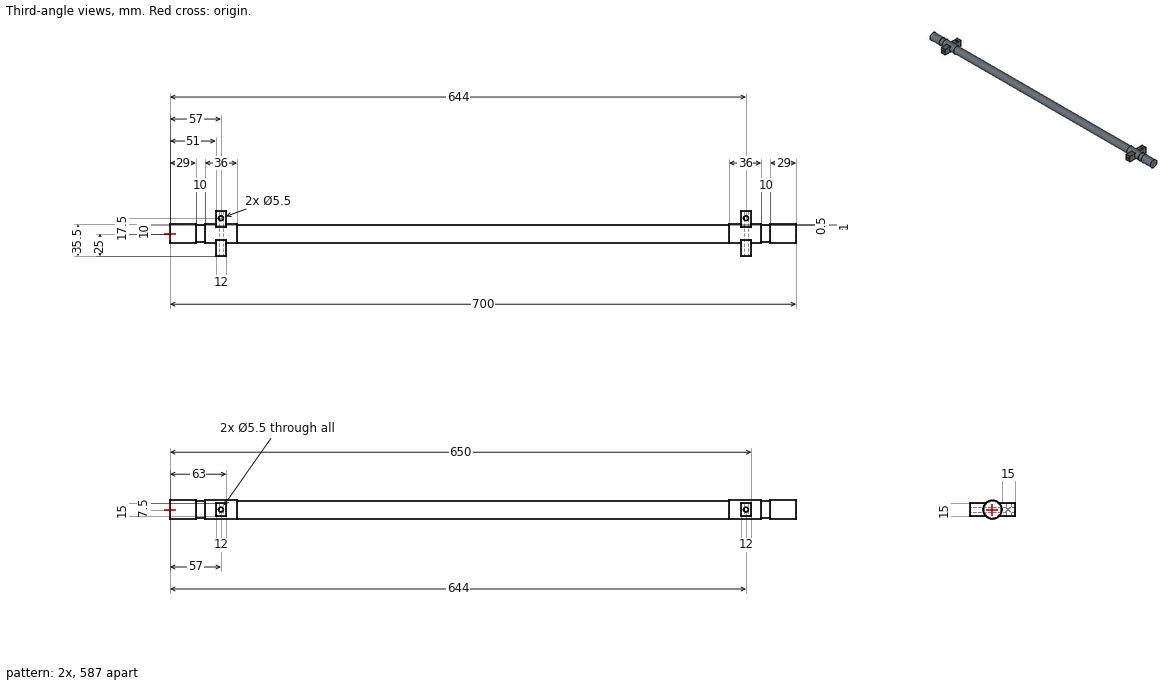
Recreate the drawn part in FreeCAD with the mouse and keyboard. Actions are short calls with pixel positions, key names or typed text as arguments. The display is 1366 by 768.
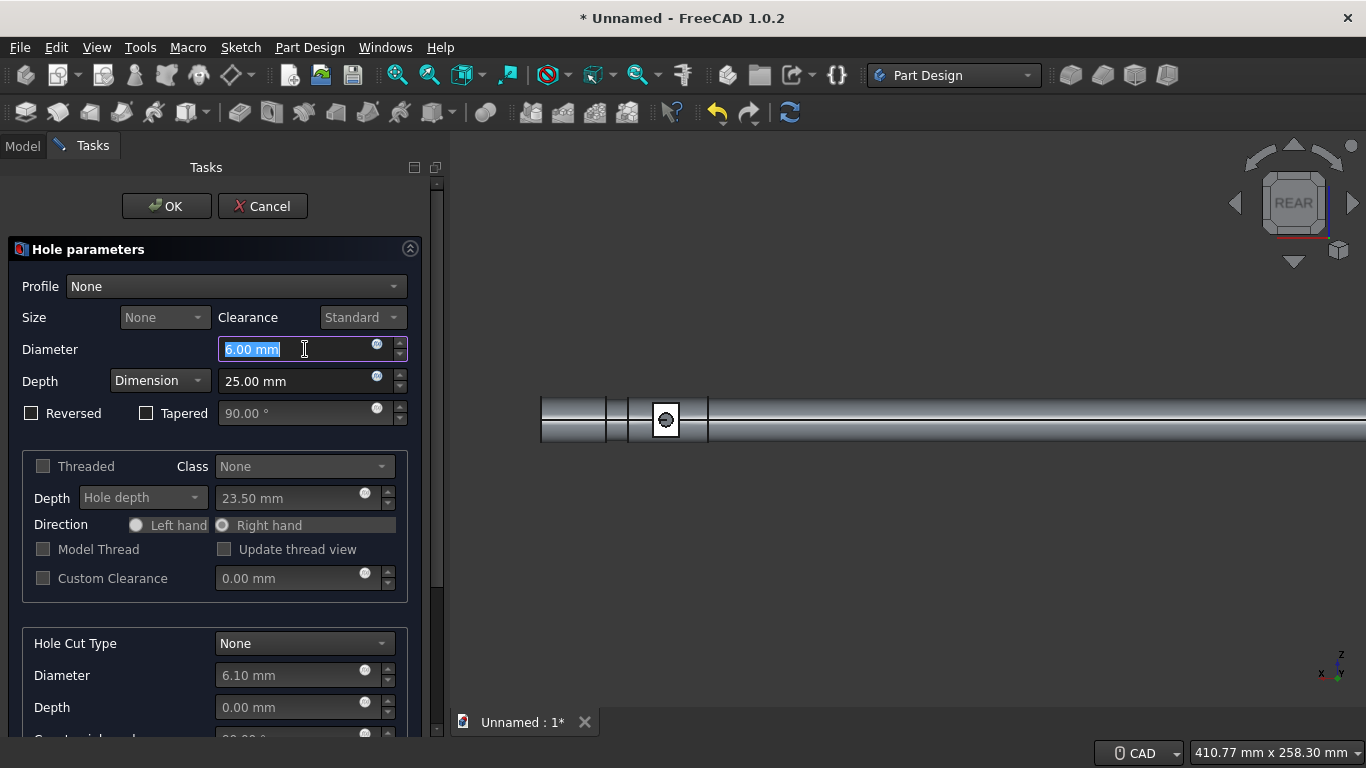
text(5.5)
key(Tab)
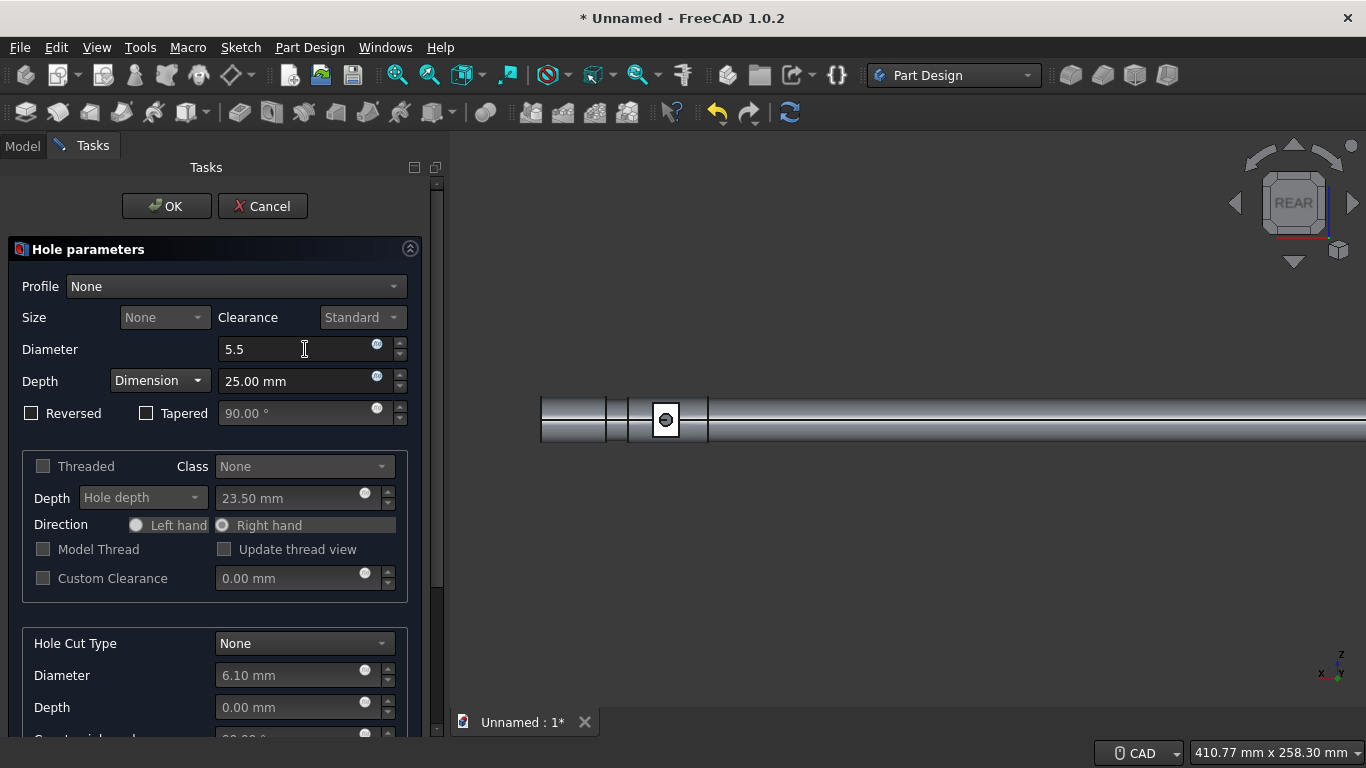
click(161, 380)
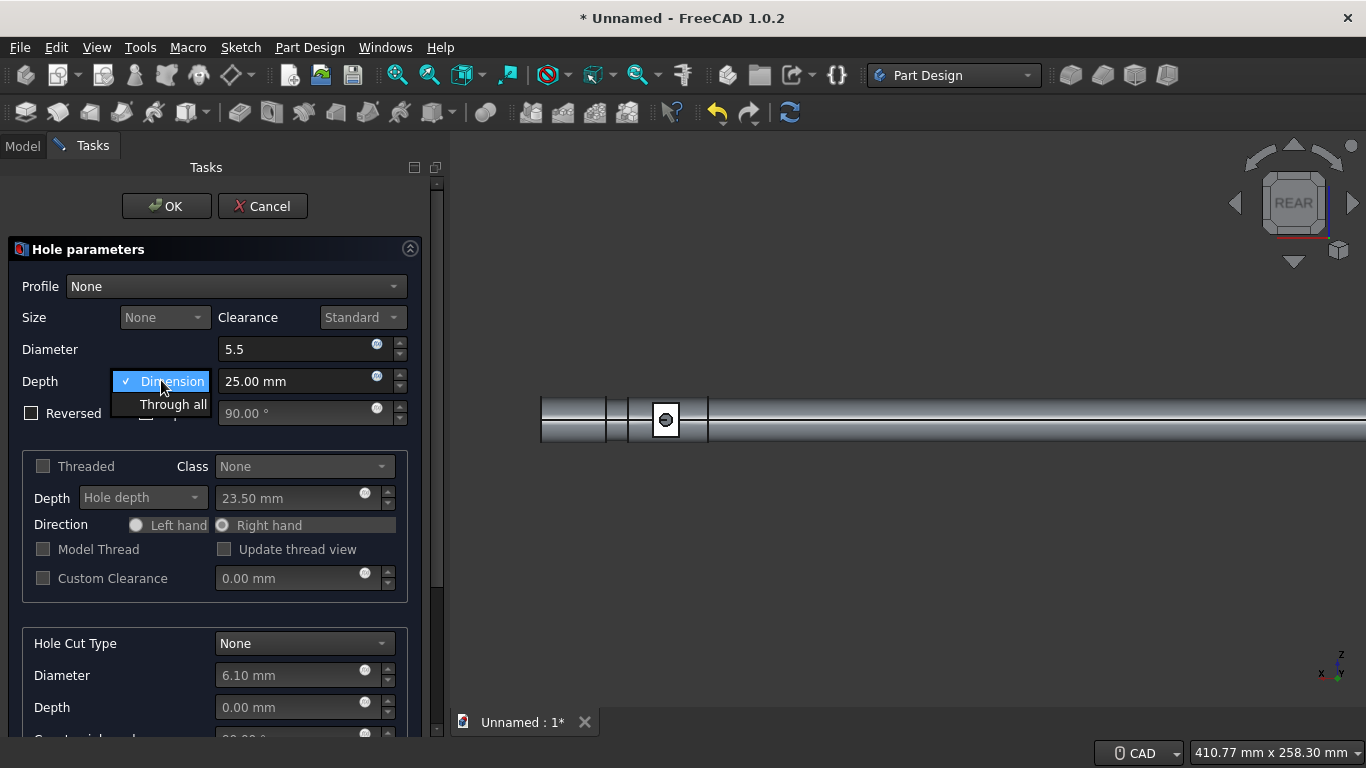
click(160, 404)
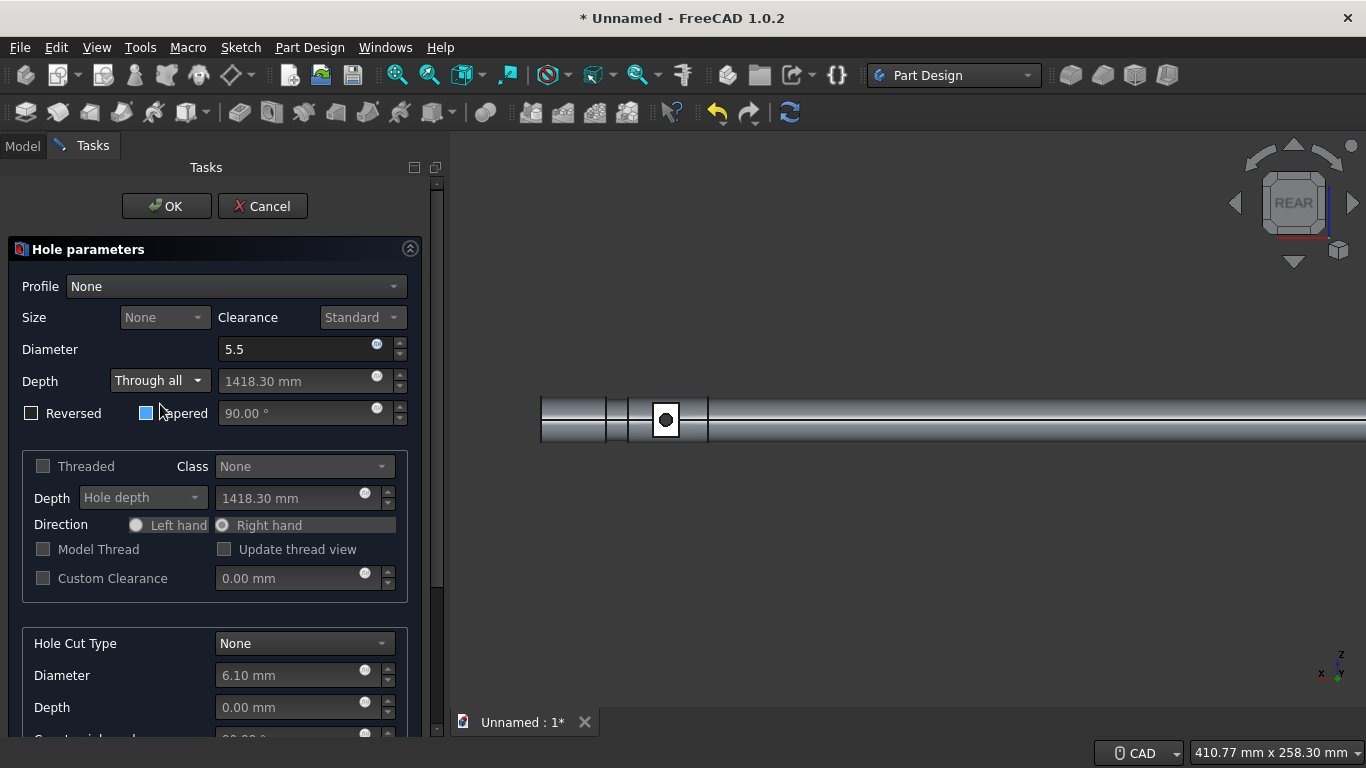
click(167, 206)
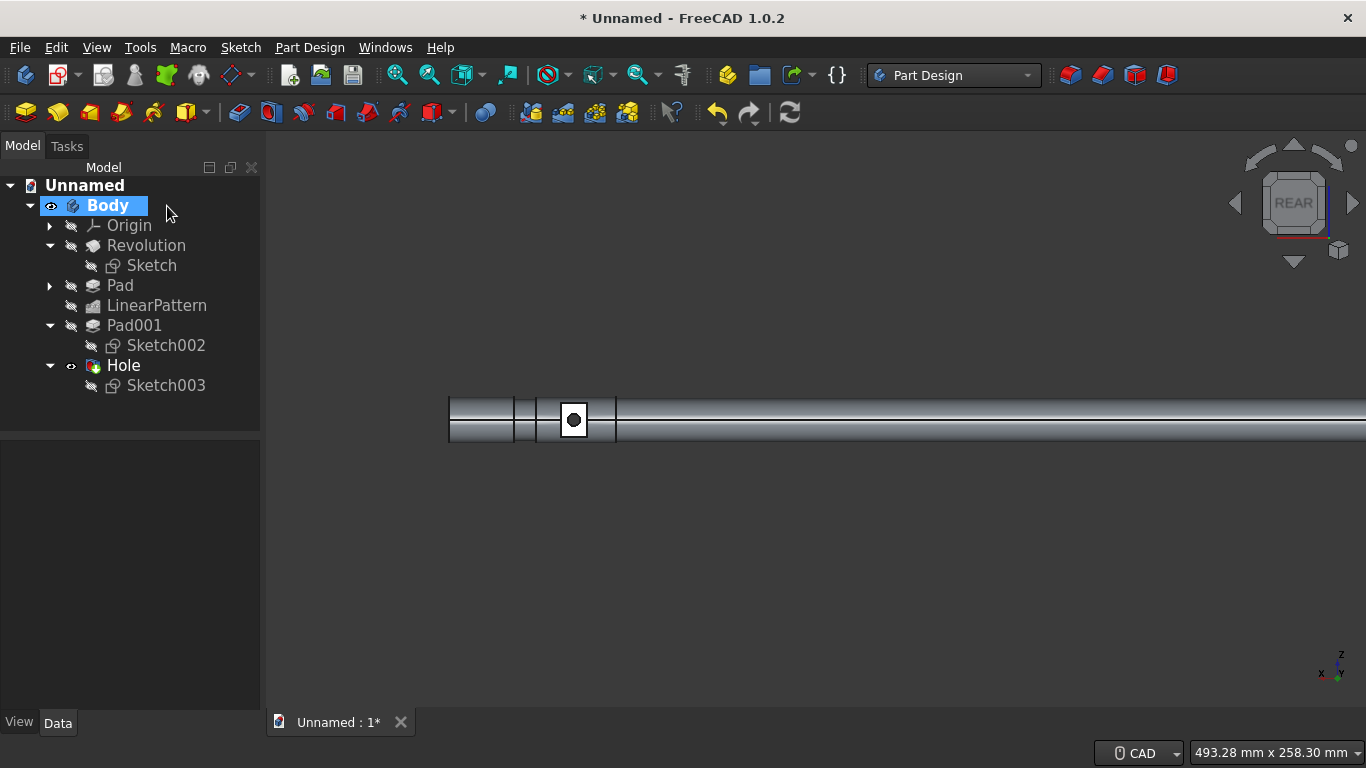
click(398, 76)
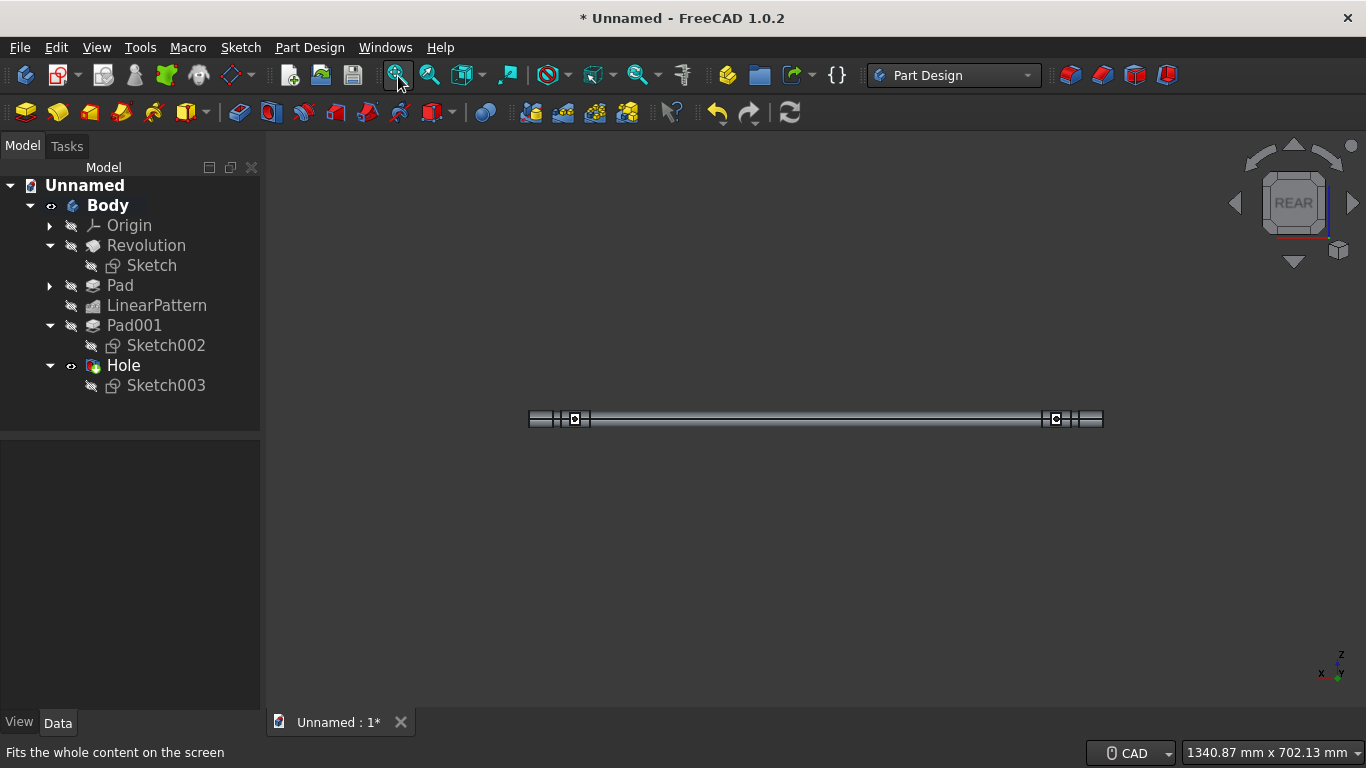
key(0)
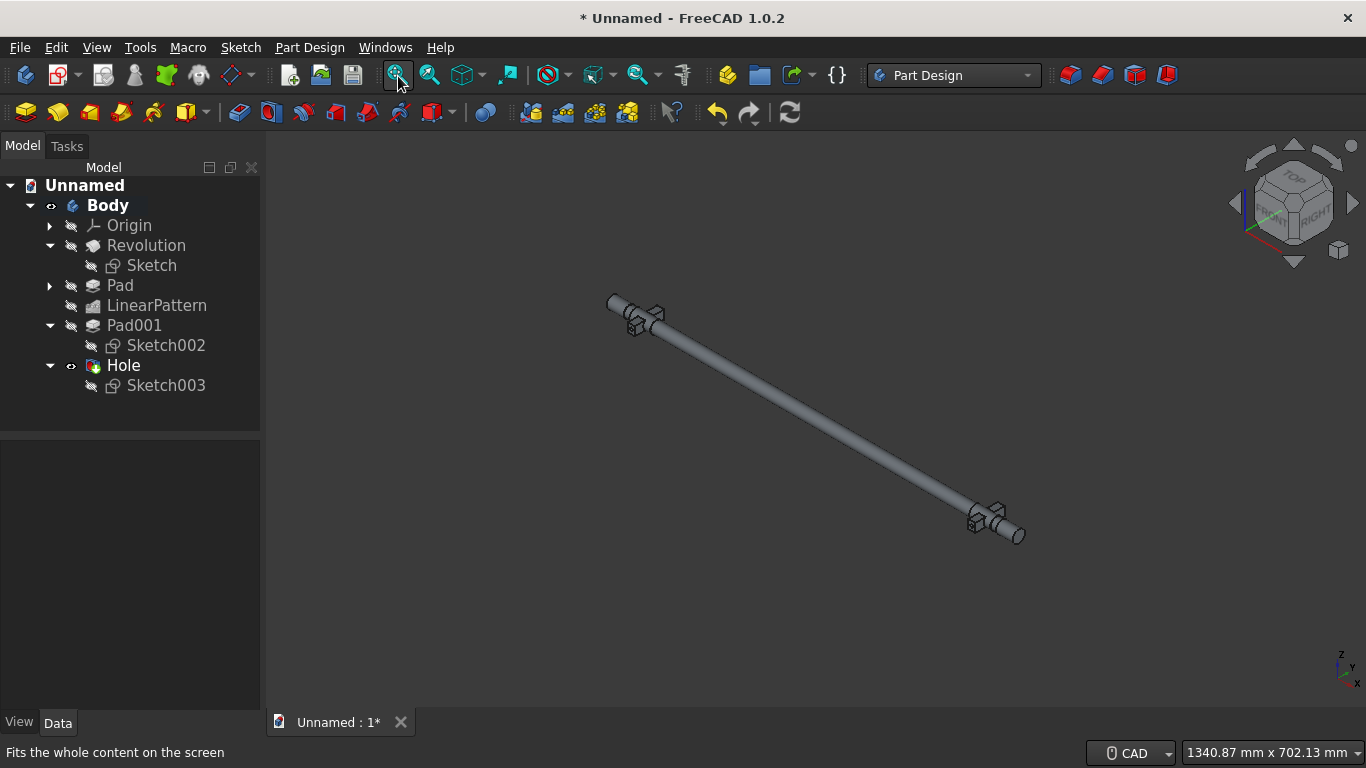
scroll(657, 309, up, 5)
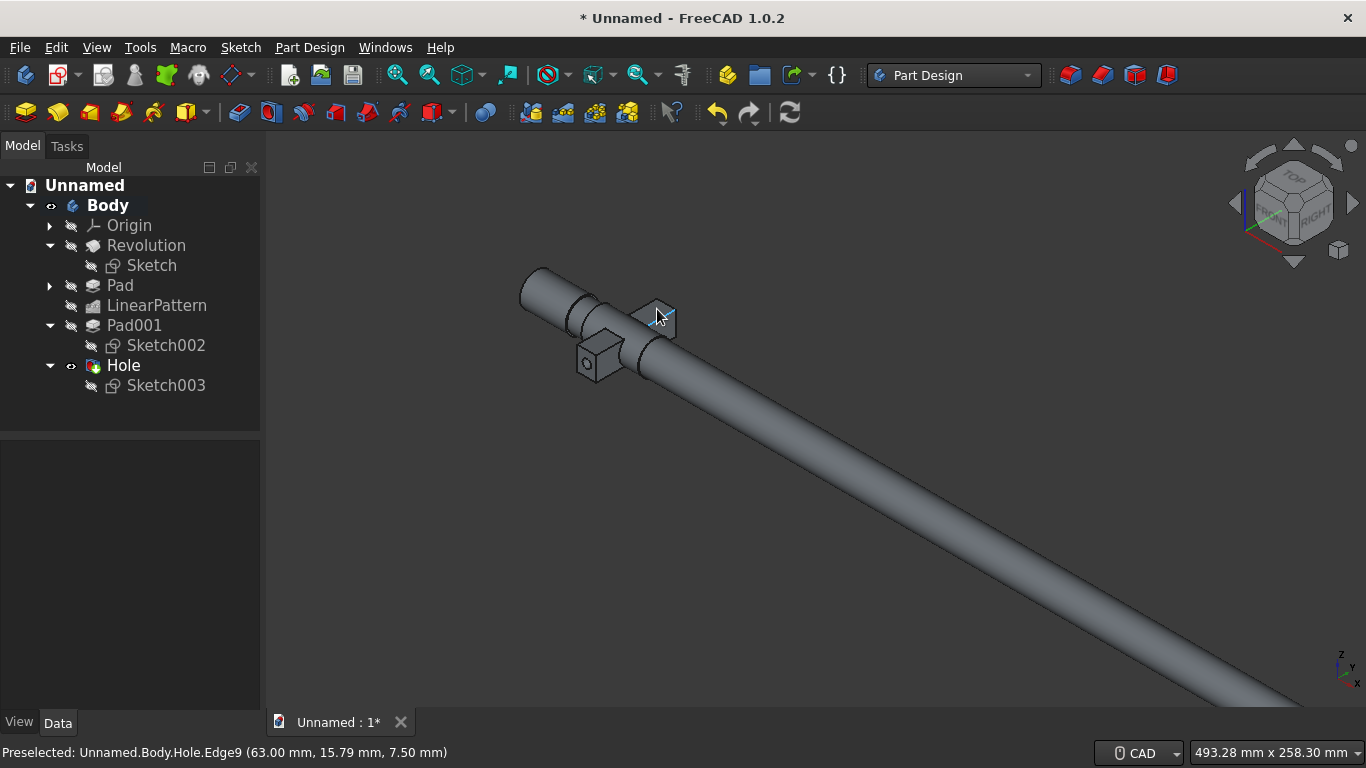
click(656, 309)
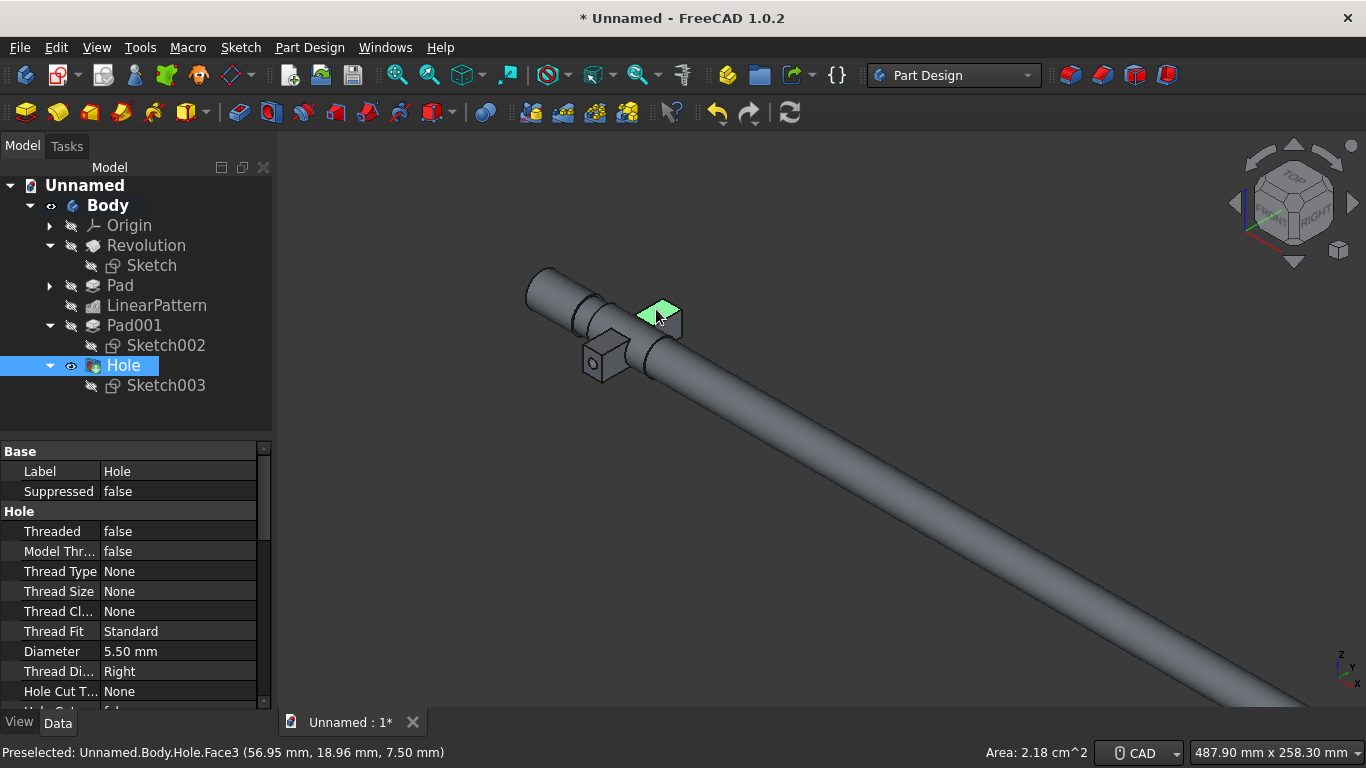
click(58, 76)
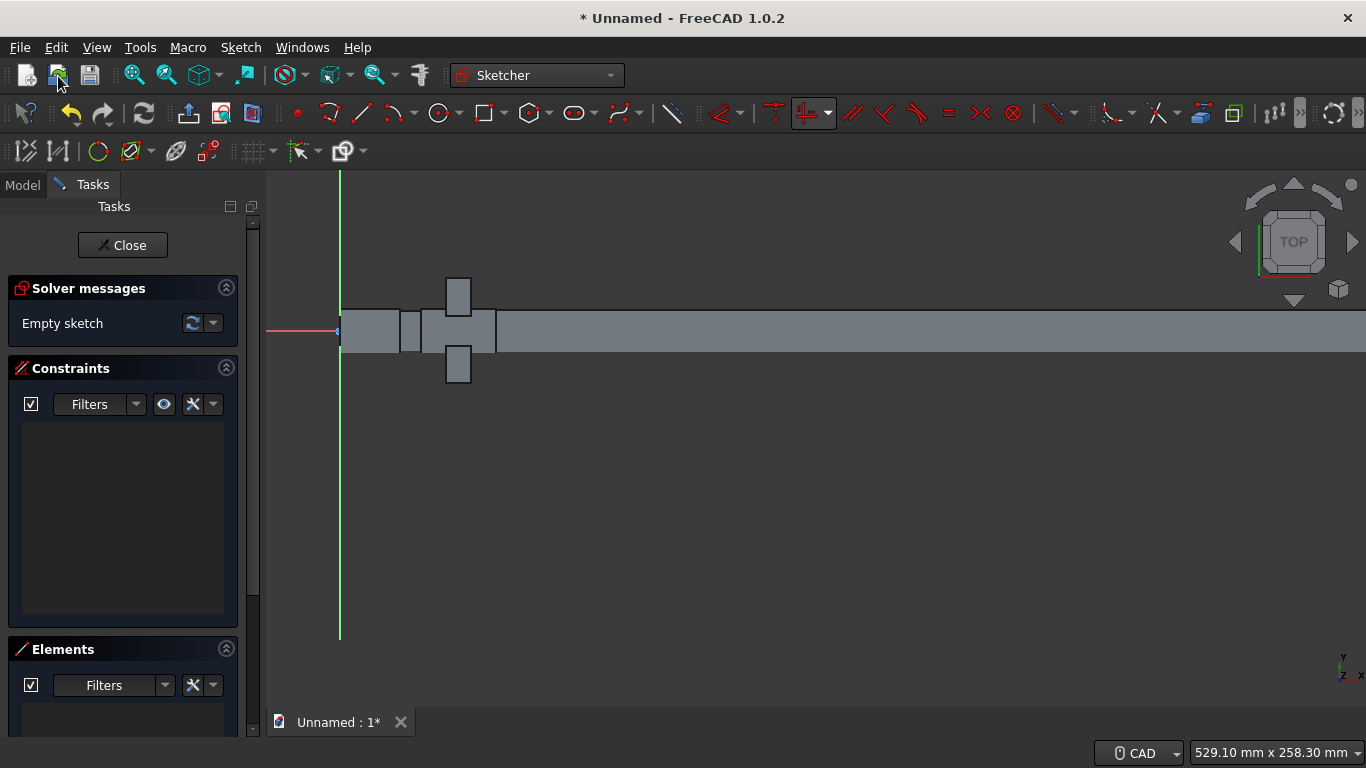
click(254, 114)